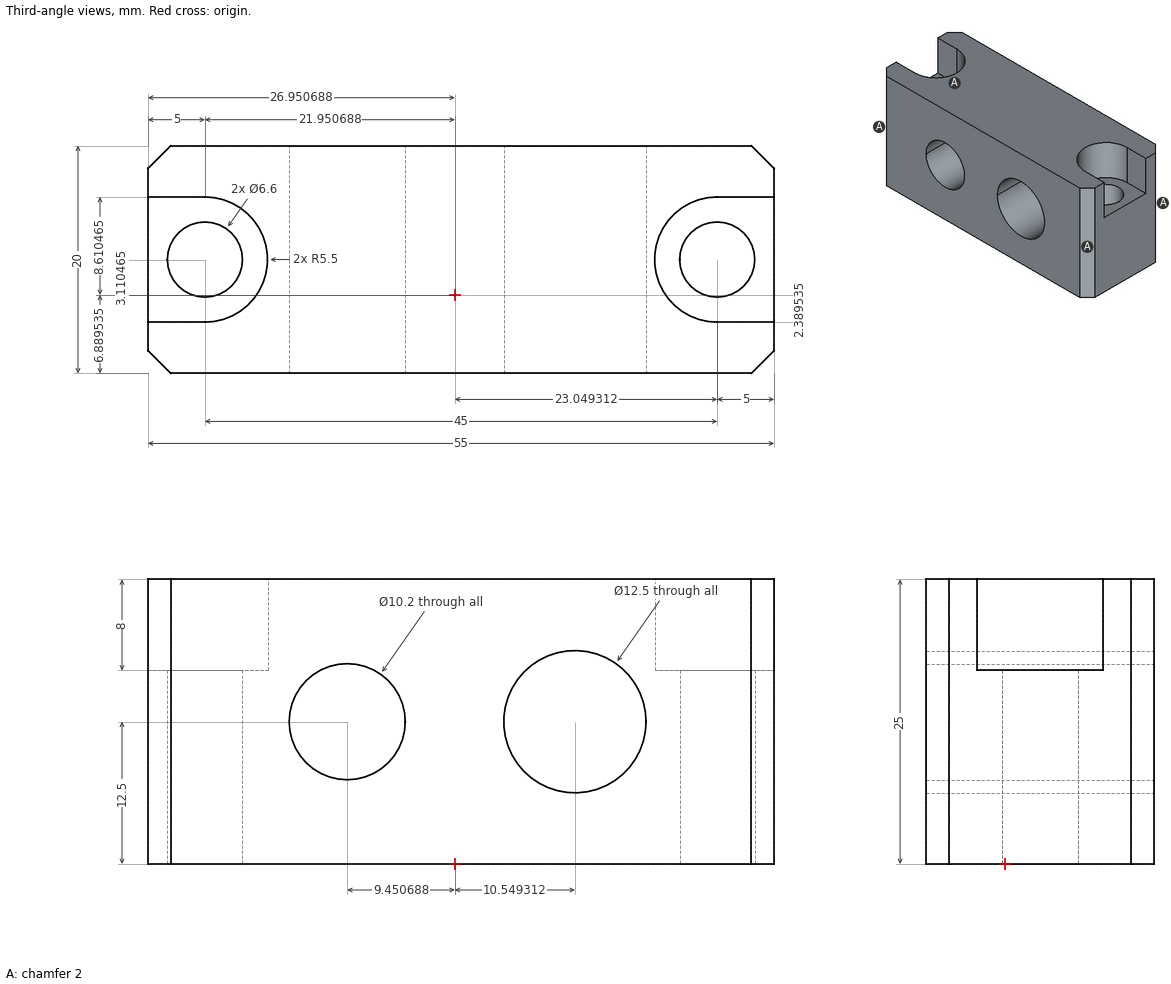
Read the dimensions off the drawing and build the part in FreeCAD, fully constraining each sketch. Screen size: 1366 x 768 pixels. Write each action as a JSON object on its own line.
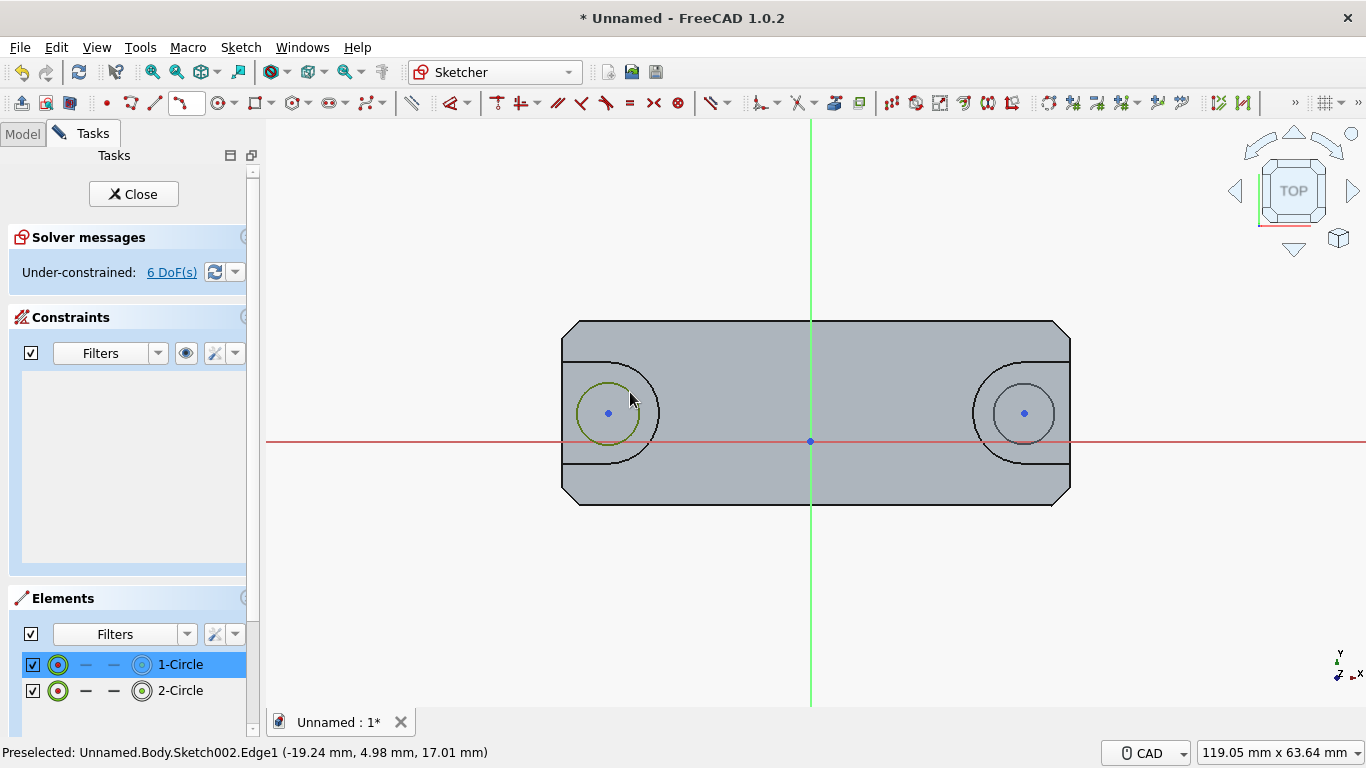
{"action": "left_click", "coordinate": [1045, 392]}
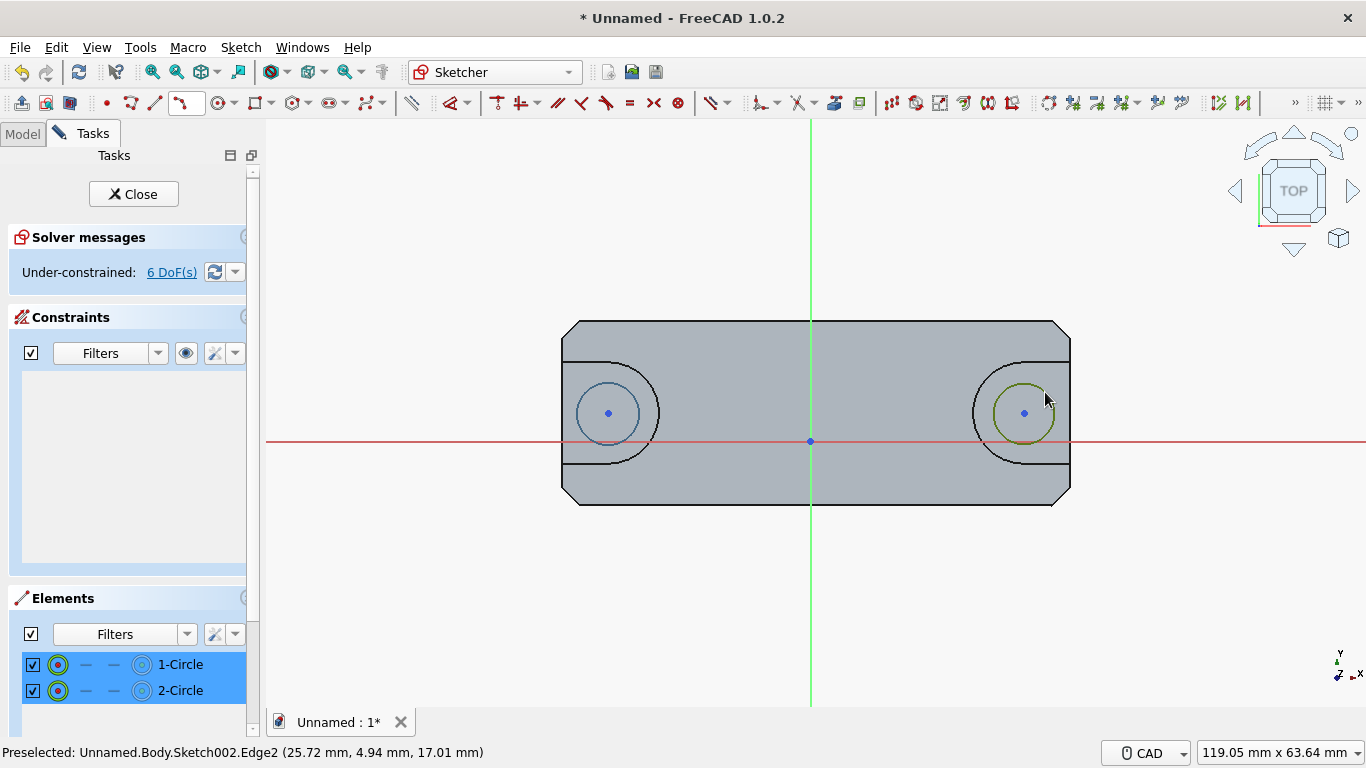
{"action": "left_click", "coordinate": [630, 104]}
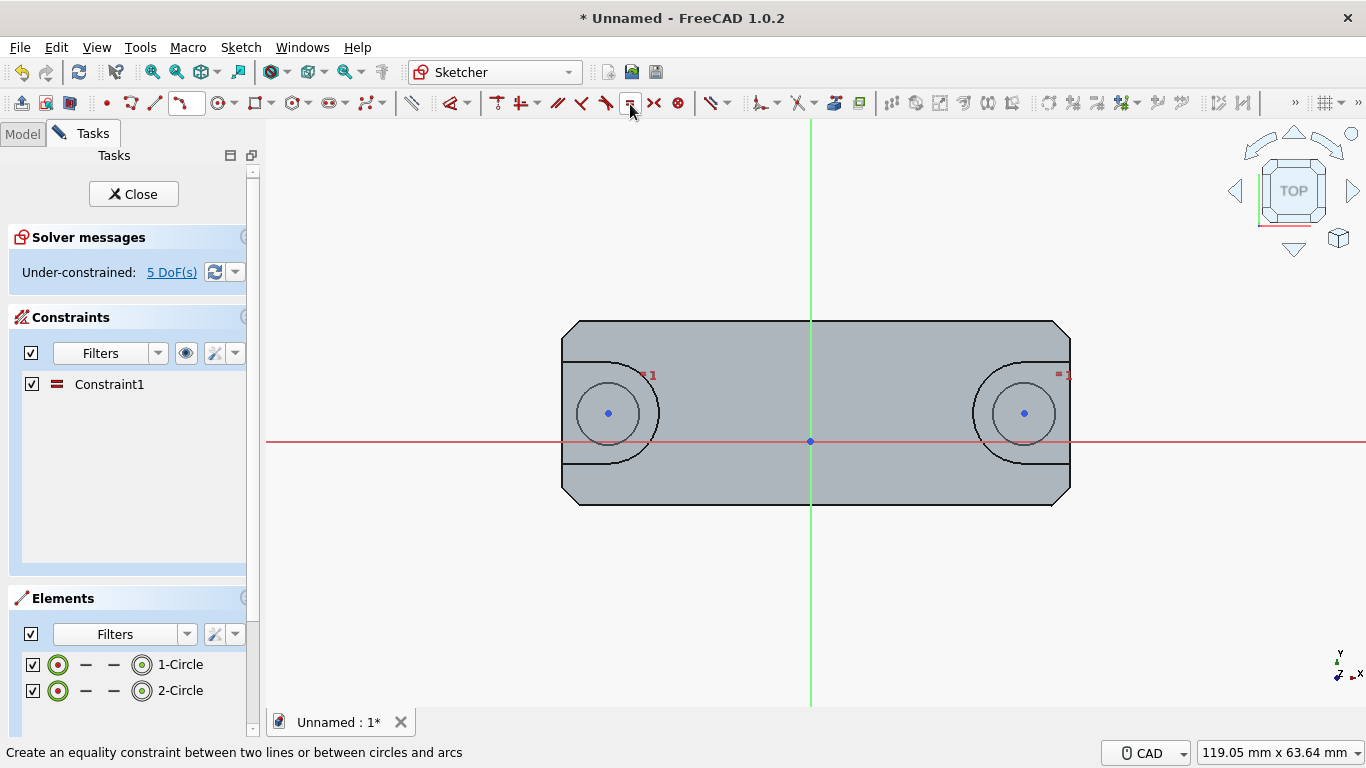
{"action": "left_click", "coordinate": [608, 414]}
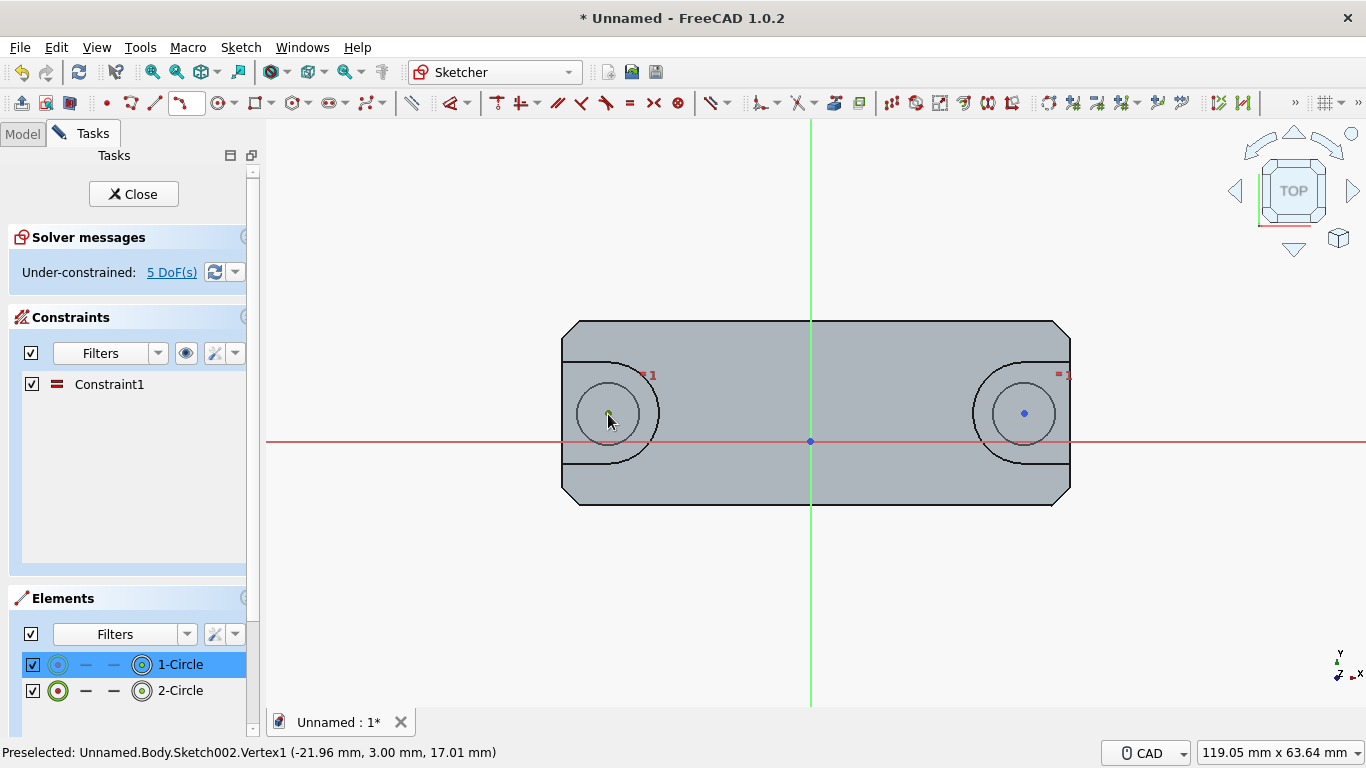
{"action": "left_click", "coordinate": [1024, 414]}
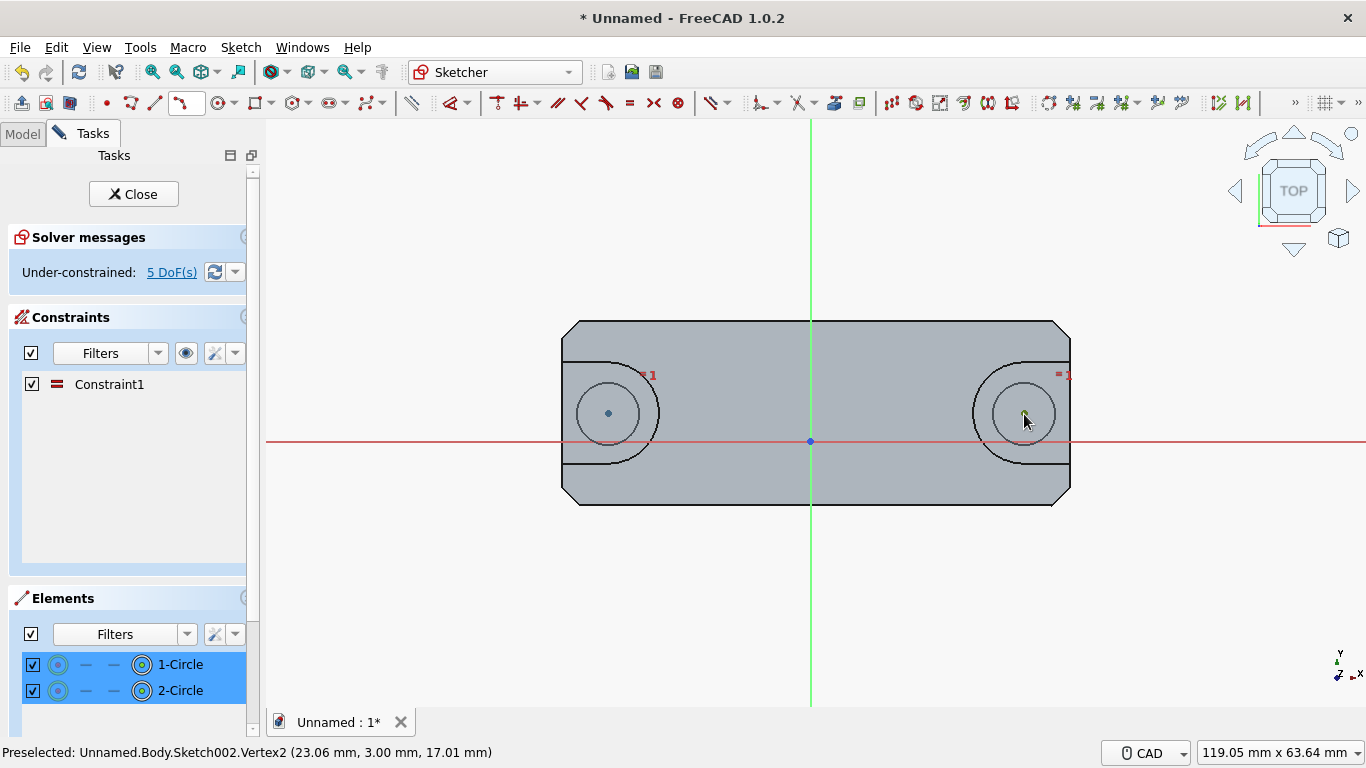
{"action": "key", "text": "h"}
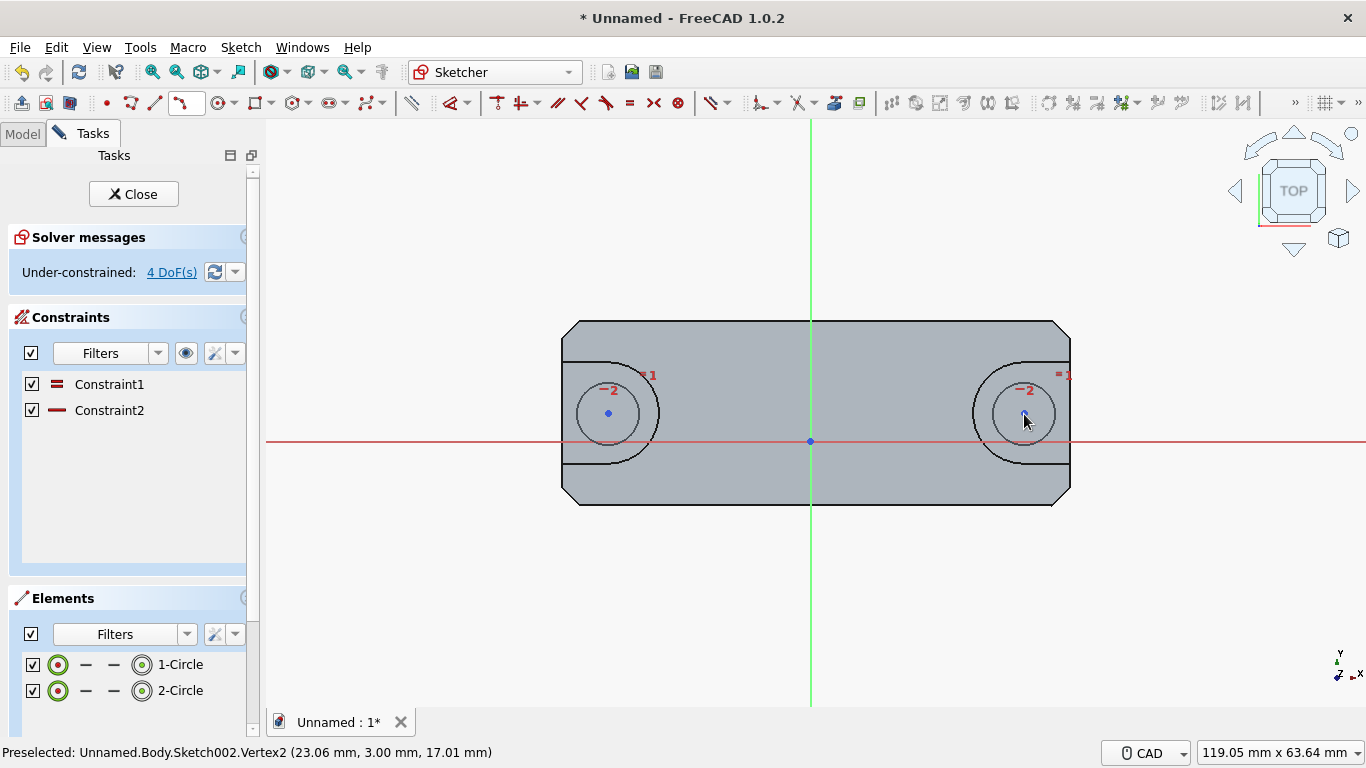
{"action": "left_click", "coordinate": [450, 104]}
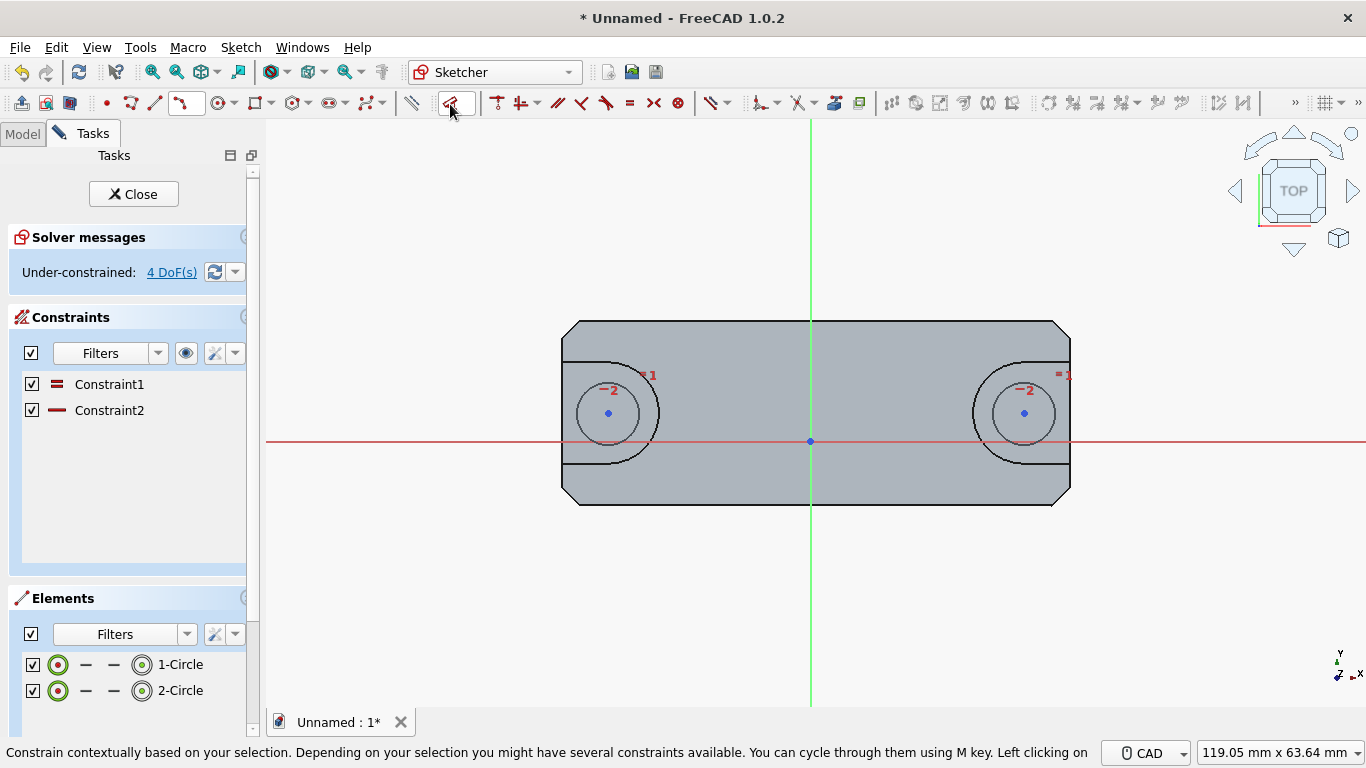
{"action": "left_click", "coordinate": [630, 392]}
{"action": "left_click", "coordinate": [653, 369]}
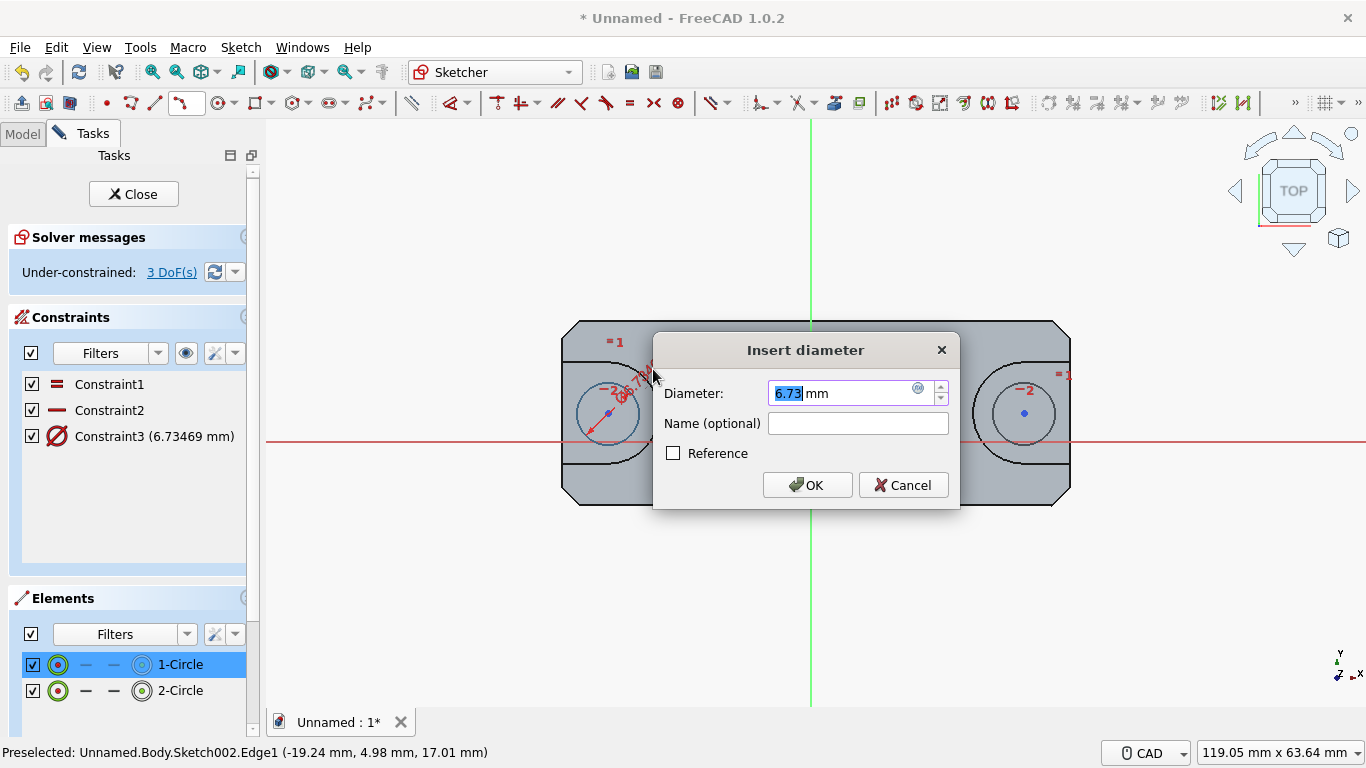
{"action": "type", "text": "6.6"}
{"action": "key", "text": "Return"}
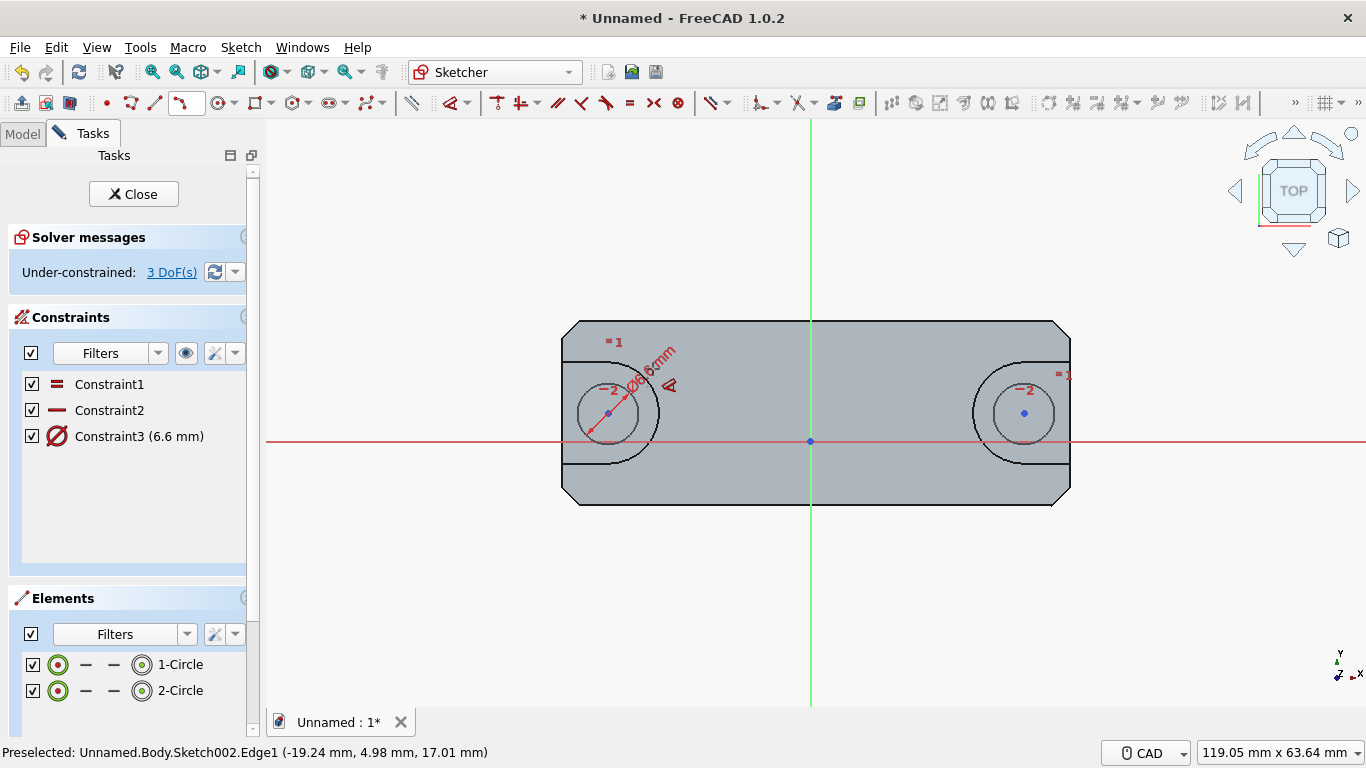
{"action": "left_click", "coordinate": [608, 414]}